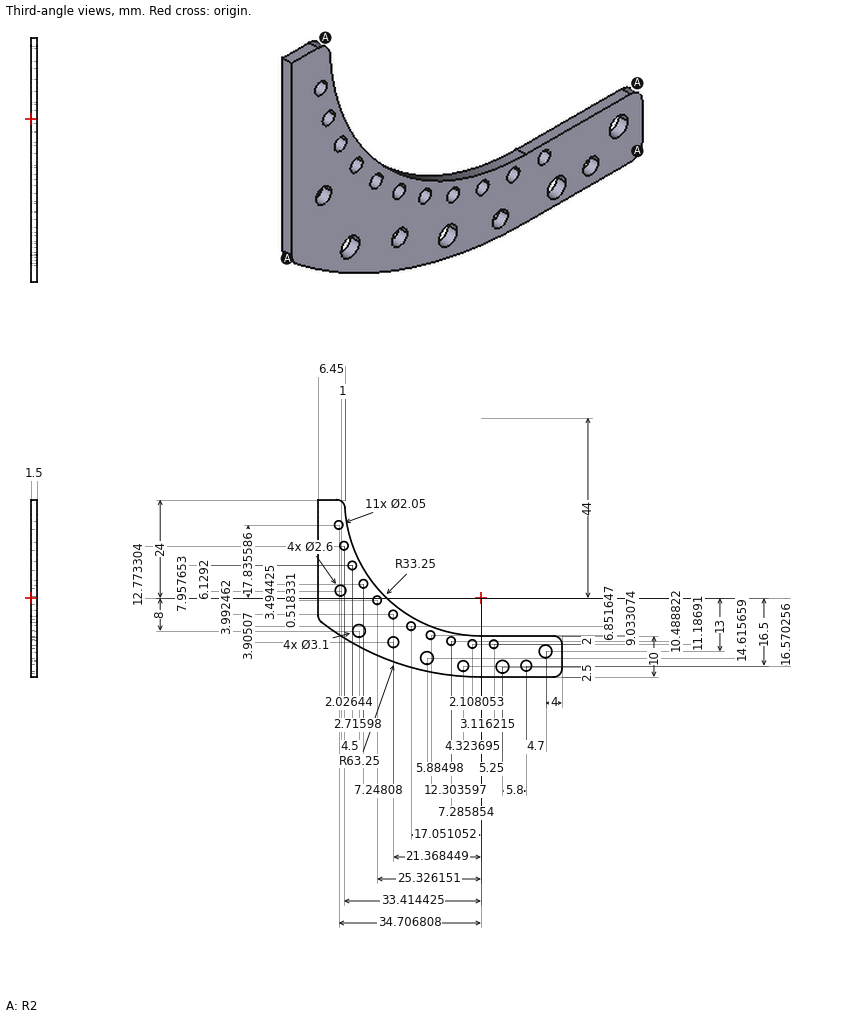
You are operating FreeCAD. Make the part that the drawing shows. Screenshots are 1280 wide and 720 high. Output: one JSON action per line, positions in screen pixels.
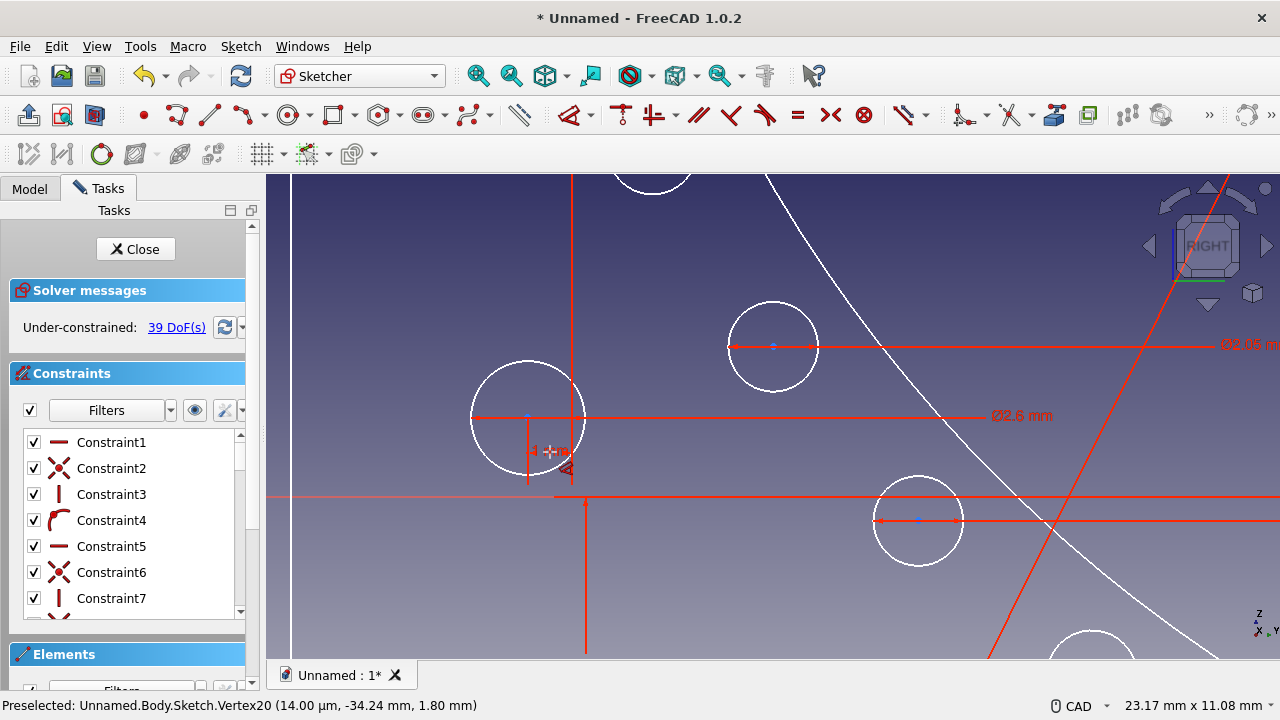
{"action": "scroll", "coordinate": [529, 421], "scroll_direction": "down", "scroll_amount": 9}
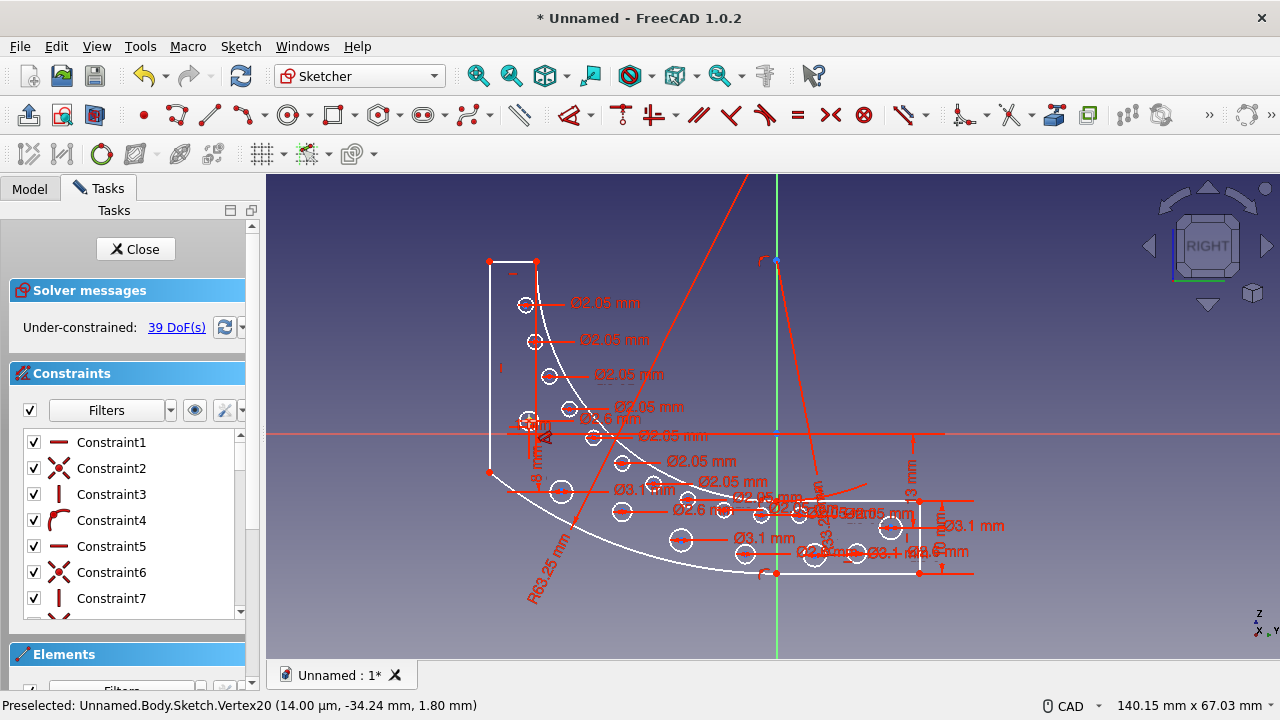
{"action": "scroll", "coordinate": [777, 501], "scroll_direction": "up", "scroll_amount": 6}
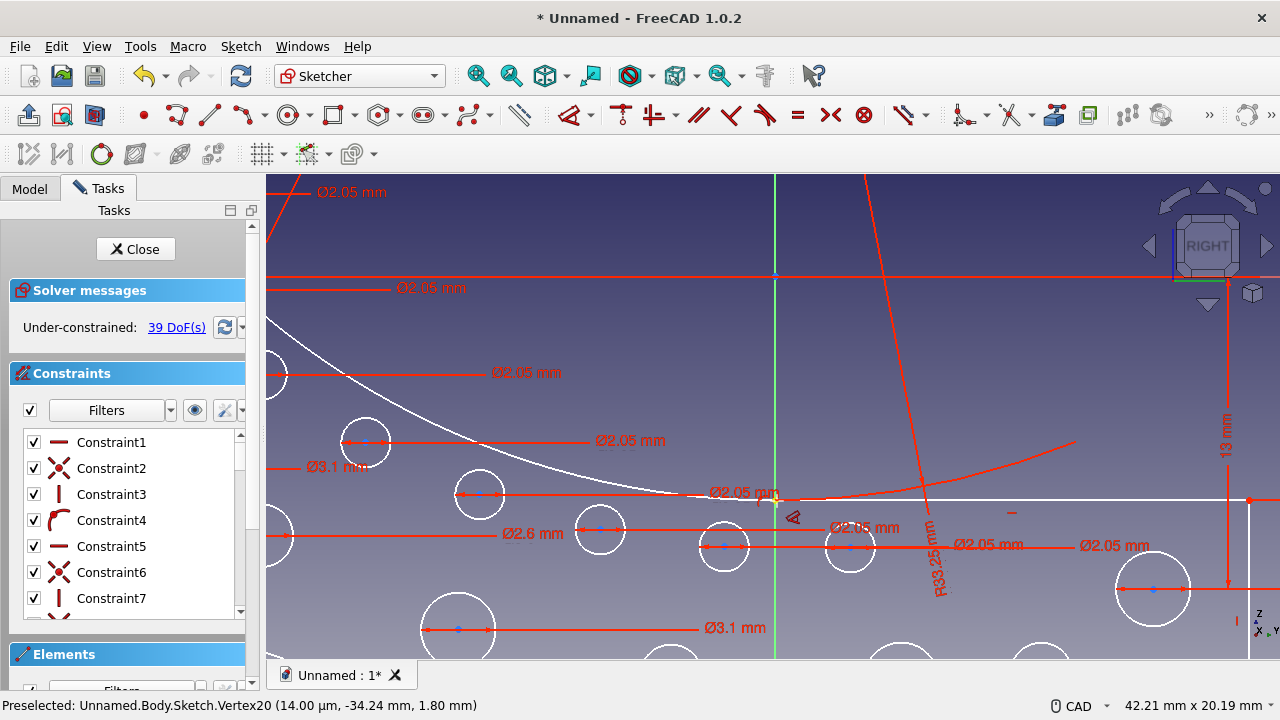
{"action": "left_click", "coordinate": [775, 500]}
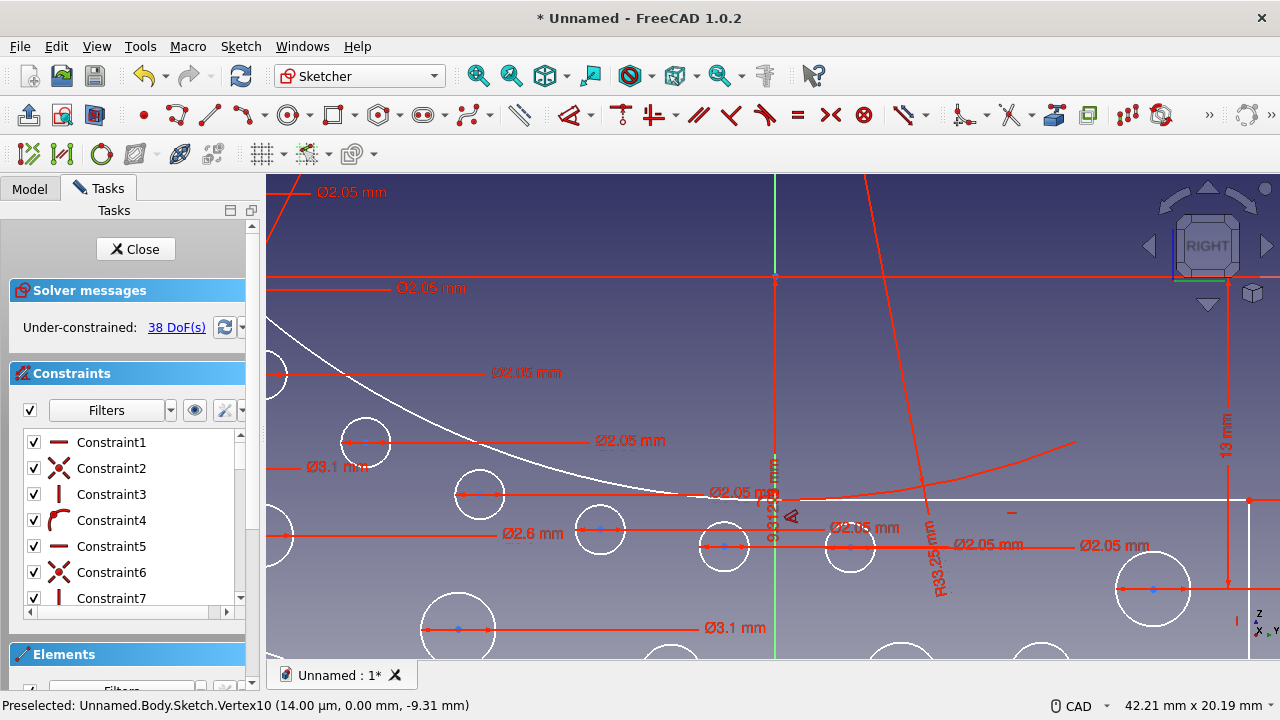
{"action": "left_click", "coordinate": [850, 548]}
{"action": "left_click", "coordinate": [884, 524]}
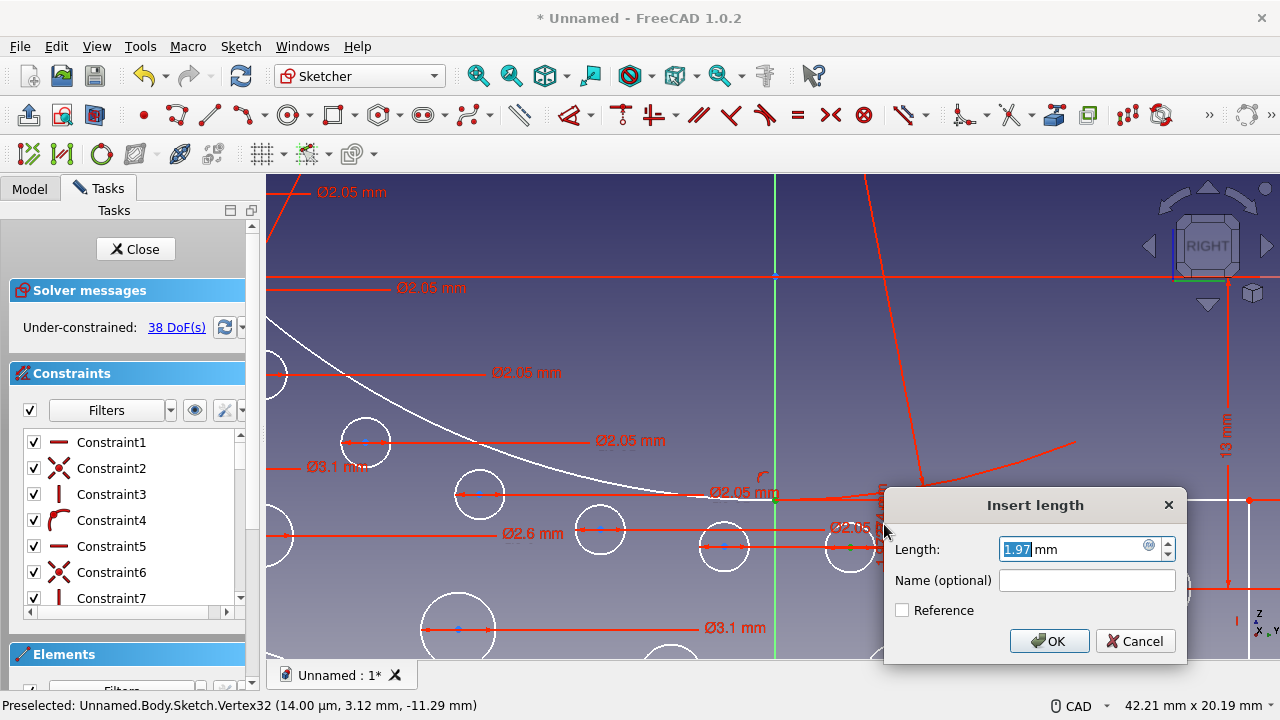
{"action": "type", "text": "2"}
{"action": "key", "text": "Return"}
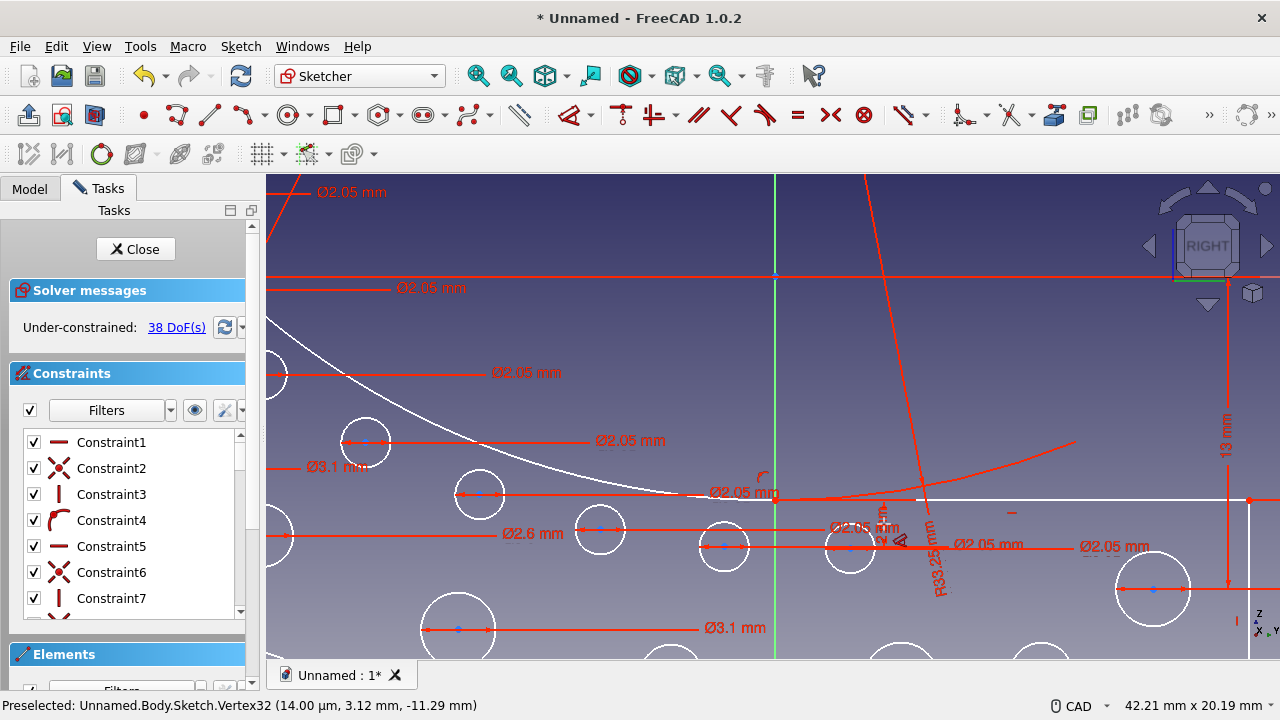
{"action": "scroll", "coordinate": [777, 501], "scroll_direction": "down", "scroll_amount": 6}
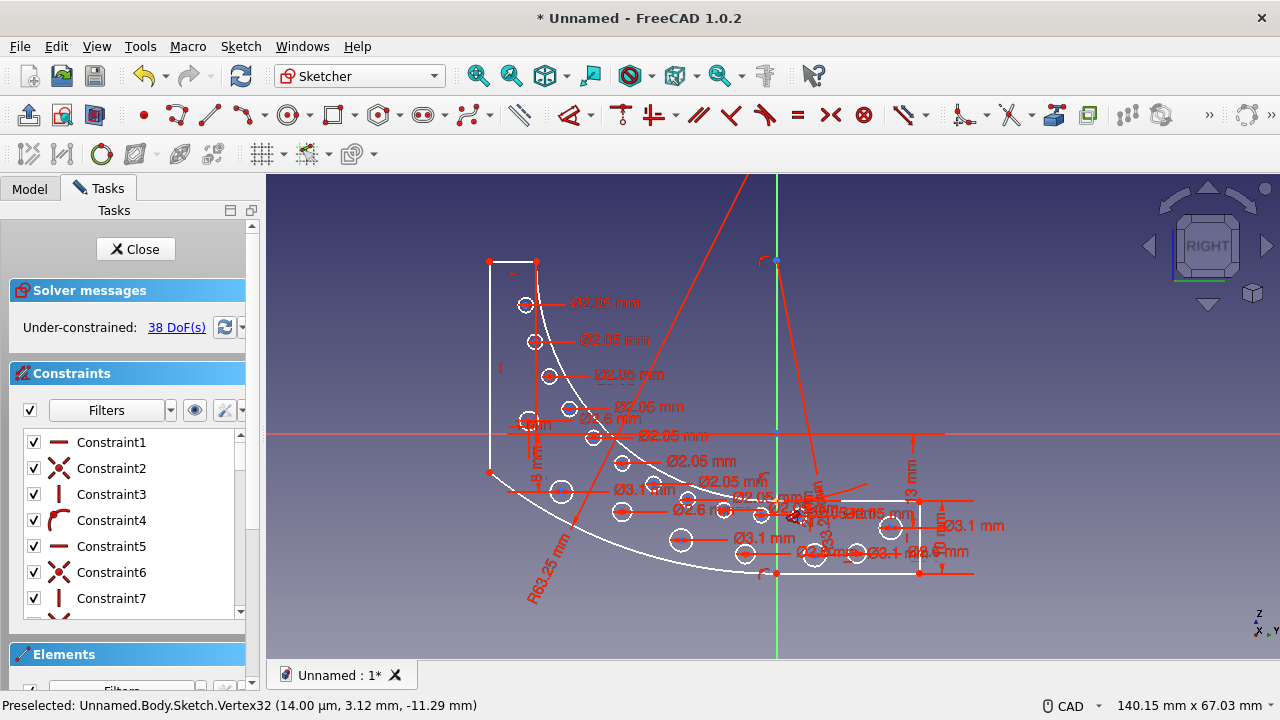
{"action": "scroll", "coordinate": [920, 501], "scroll_direction": "up", "scroll_amount": 2}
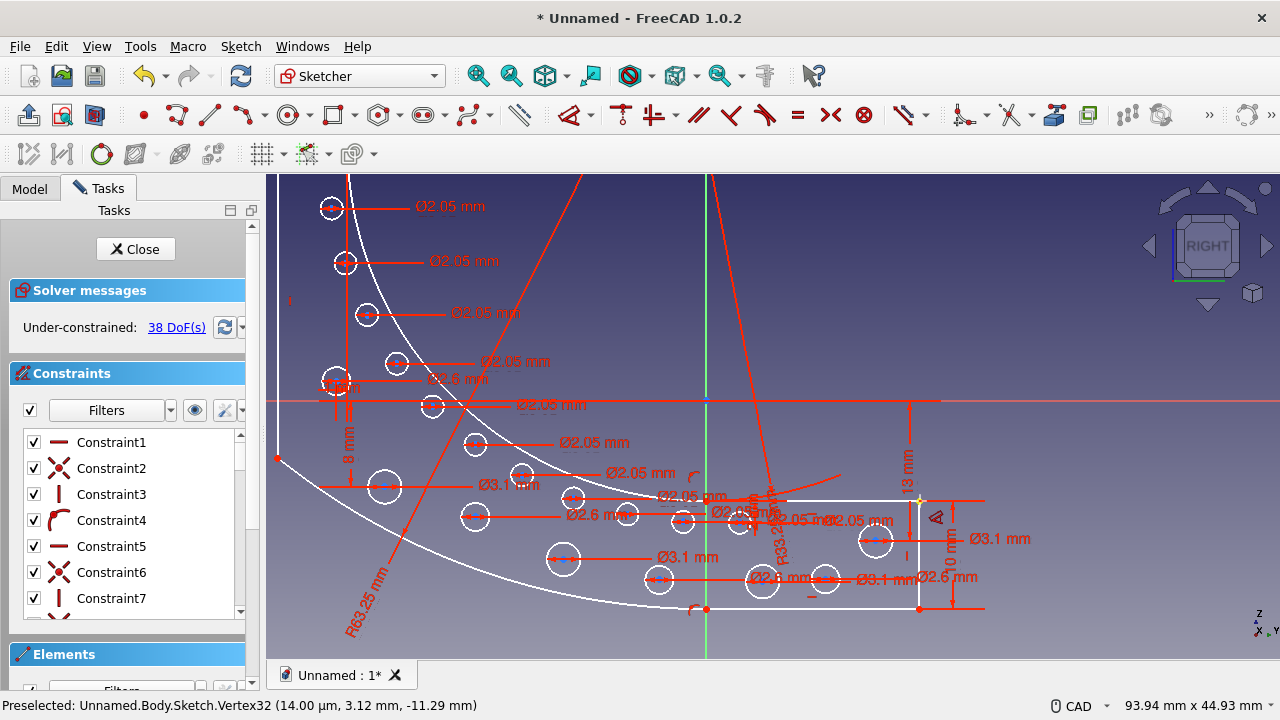
{"action": "left_click", "coordinate": [919, 501]}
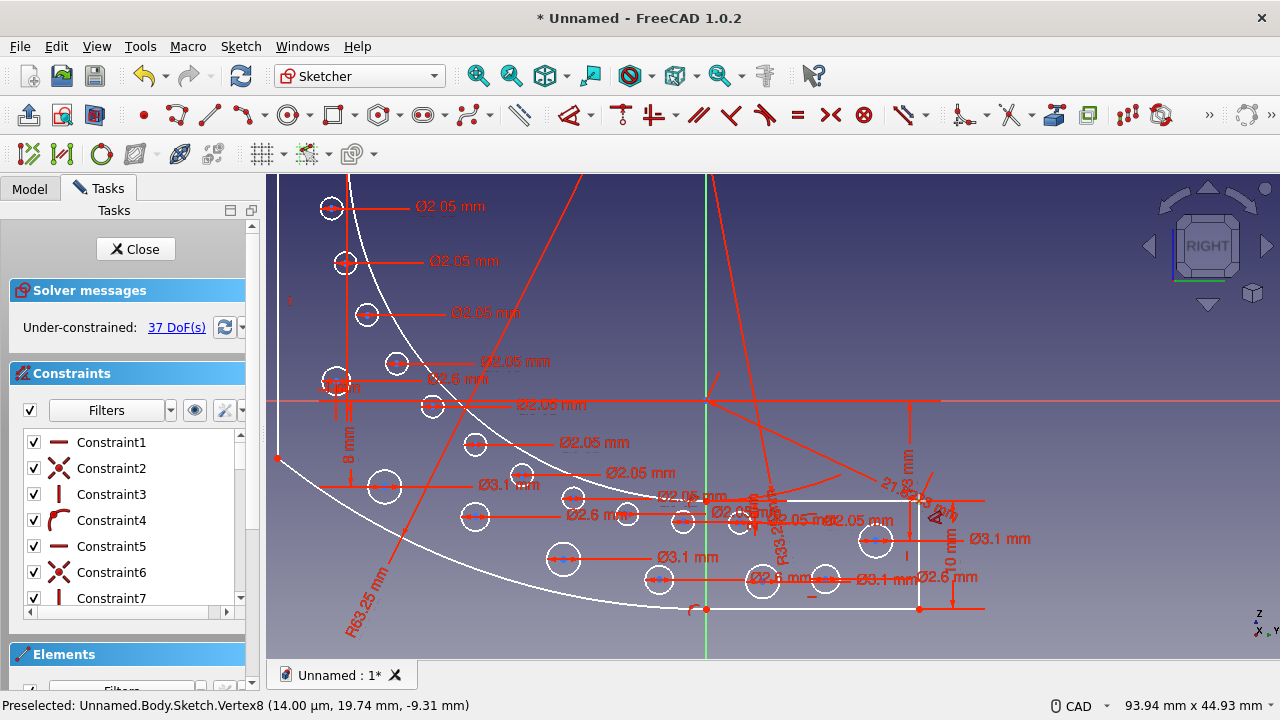
{"action": "left_click", "coordinate": [876, 541]}
{"action": "left_click", "coordinate": [898, 575]}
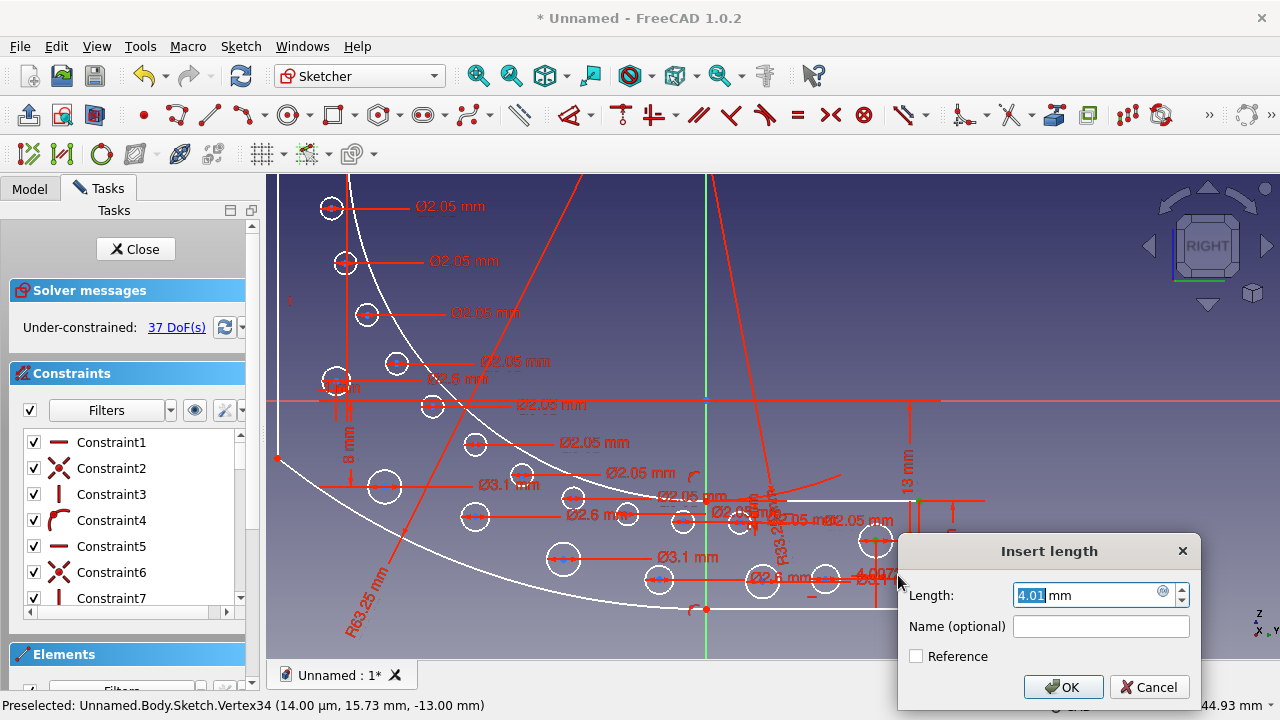
{"action": "type", "text": "4"}
{"action": "key", "text": "Return"}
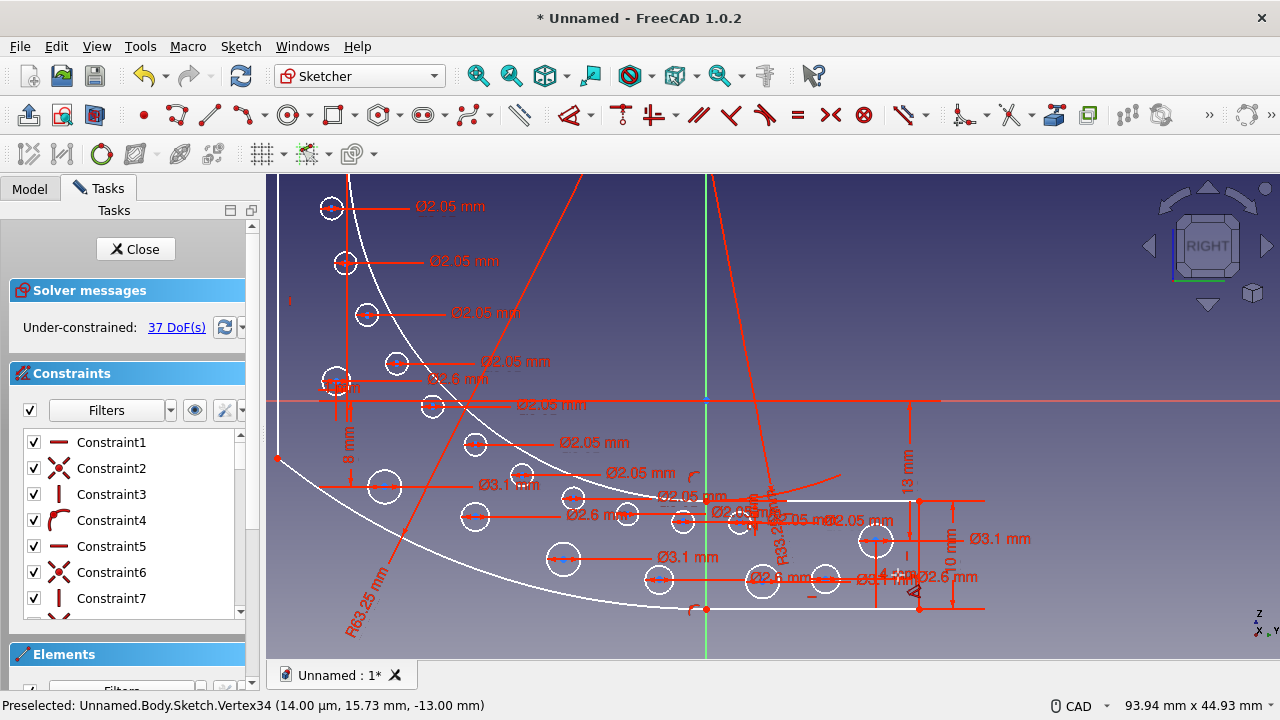
{"action": "scroll", "coordinate": [920, 501], "scroll_direction": "down", "scroll_amount": 2}